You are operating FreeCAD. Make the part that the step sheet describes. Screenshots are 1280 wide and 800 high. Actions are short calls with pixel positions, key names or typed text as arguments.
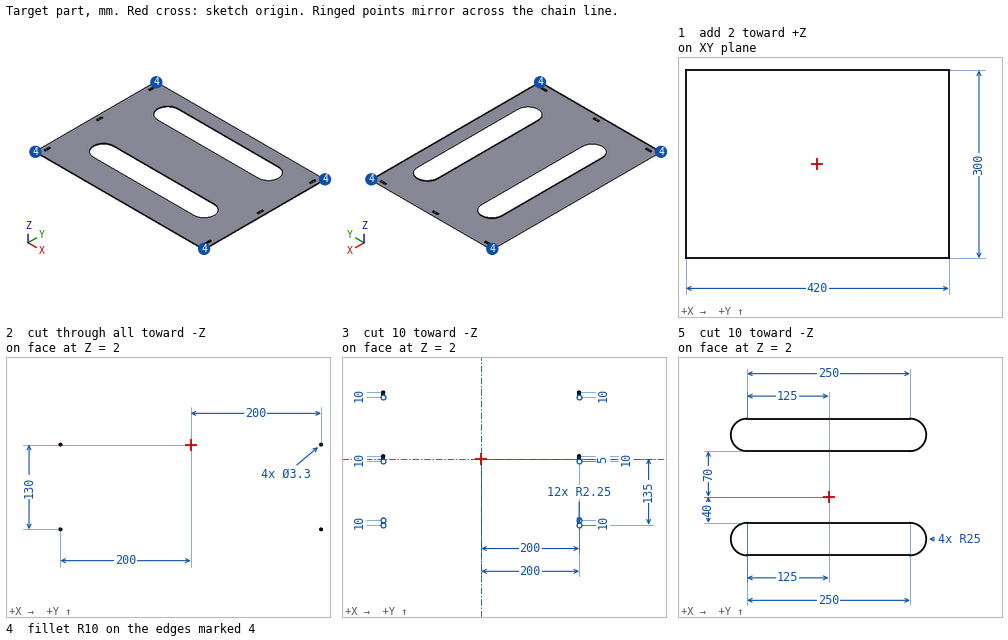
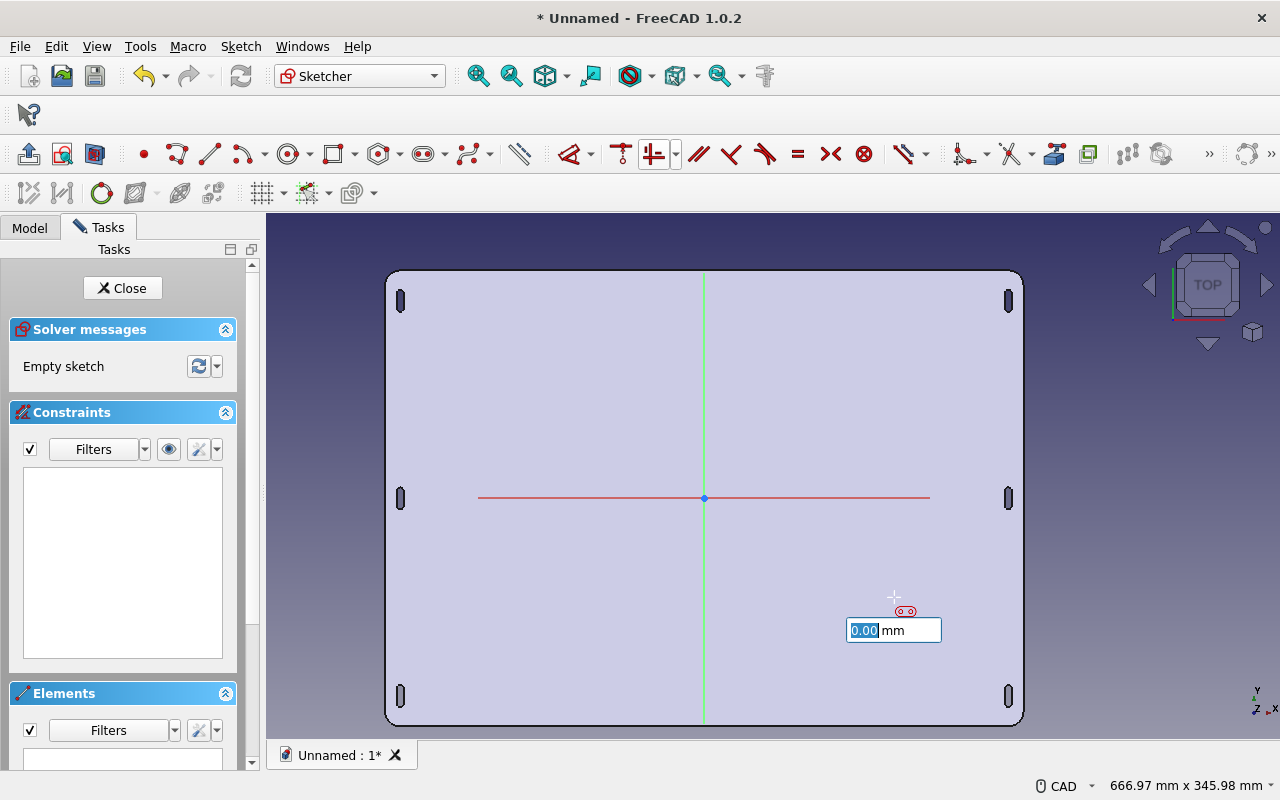
click(761, 559)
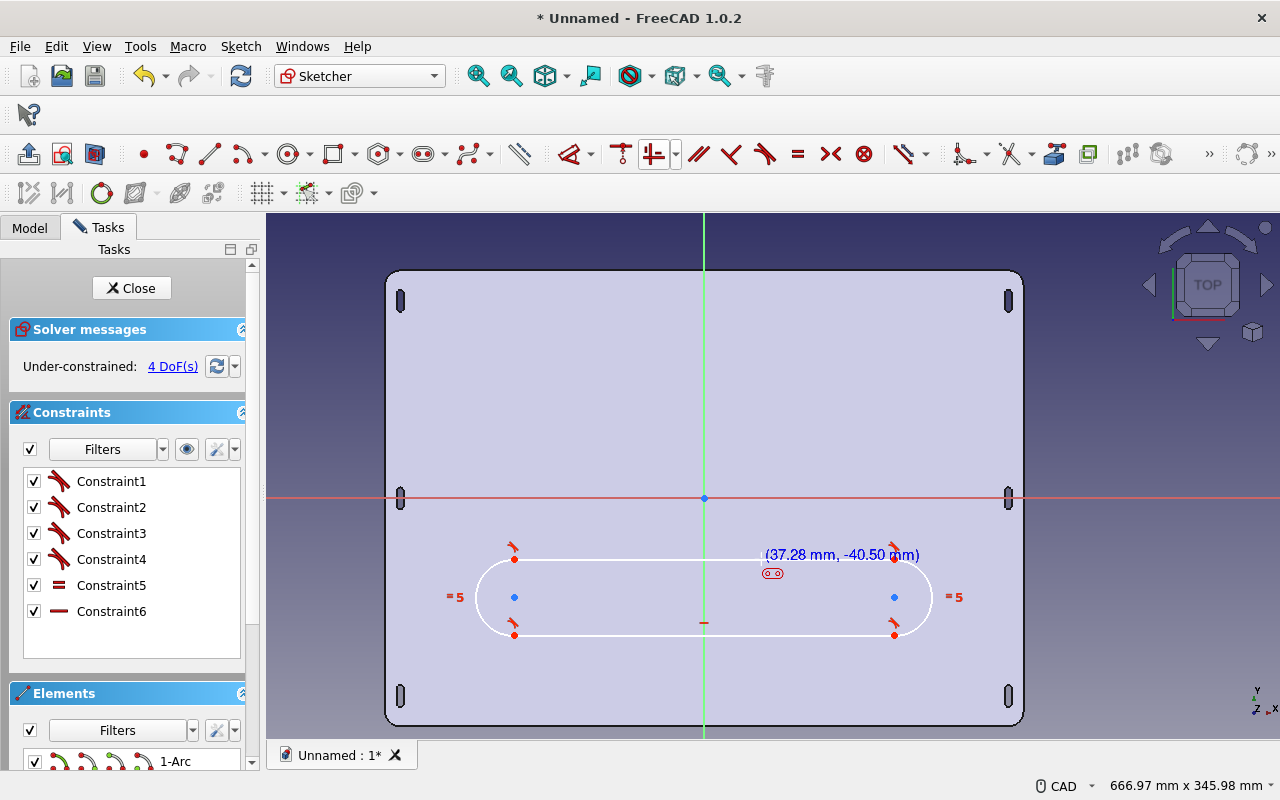
click(514, 354)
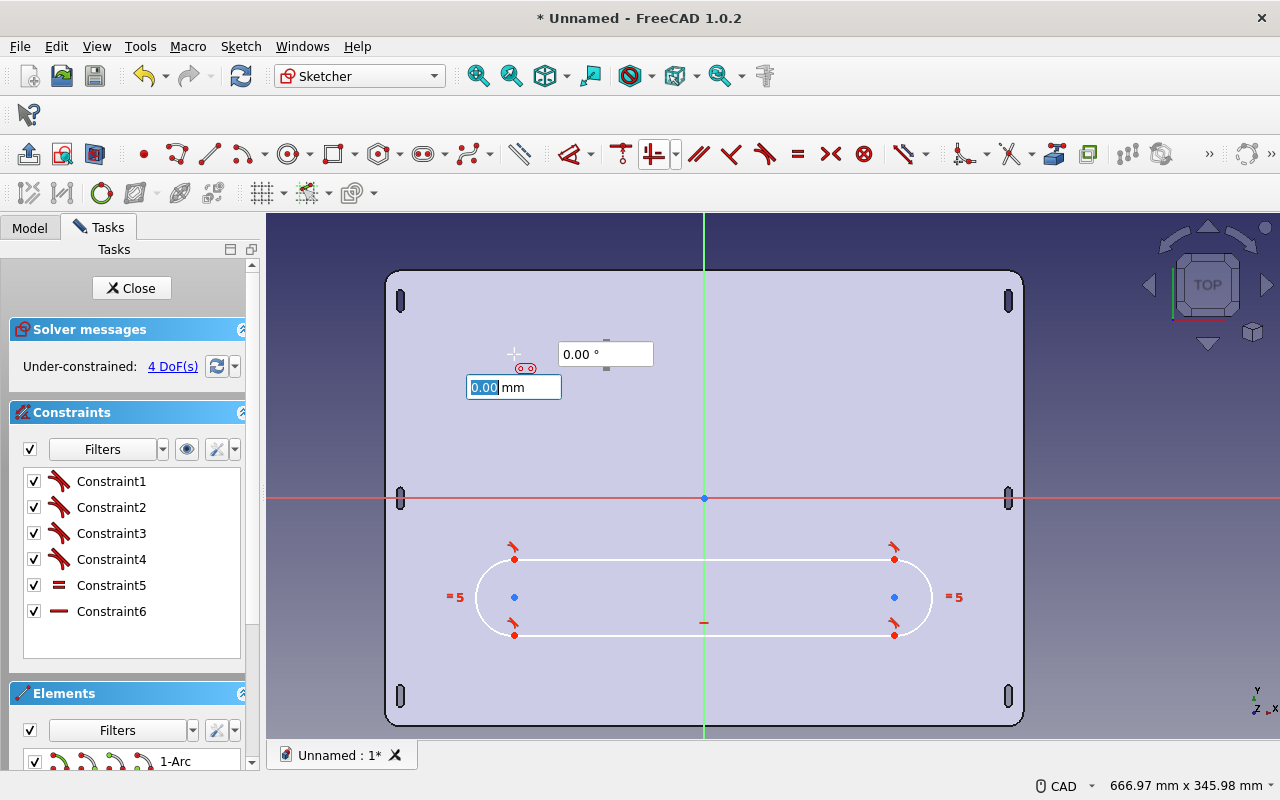
click(894, 354)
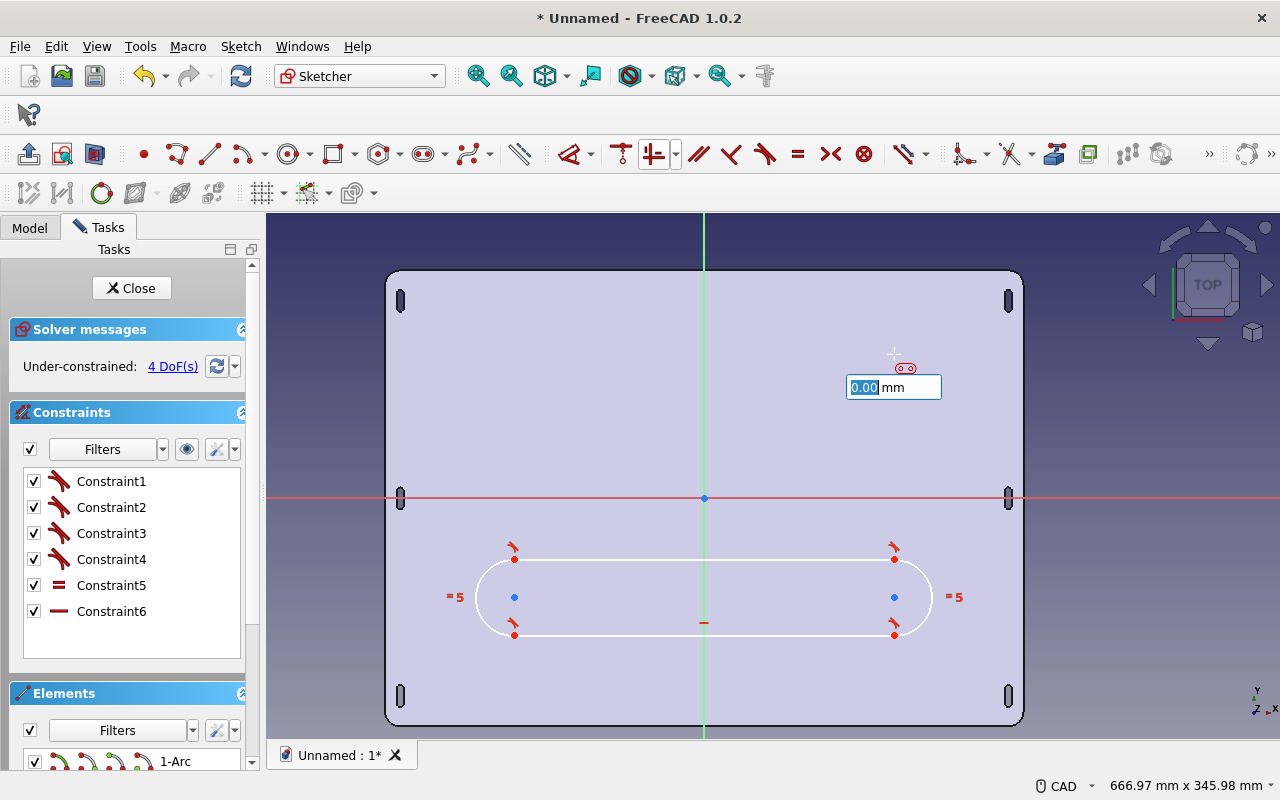
click(647, 392)
key(Escape)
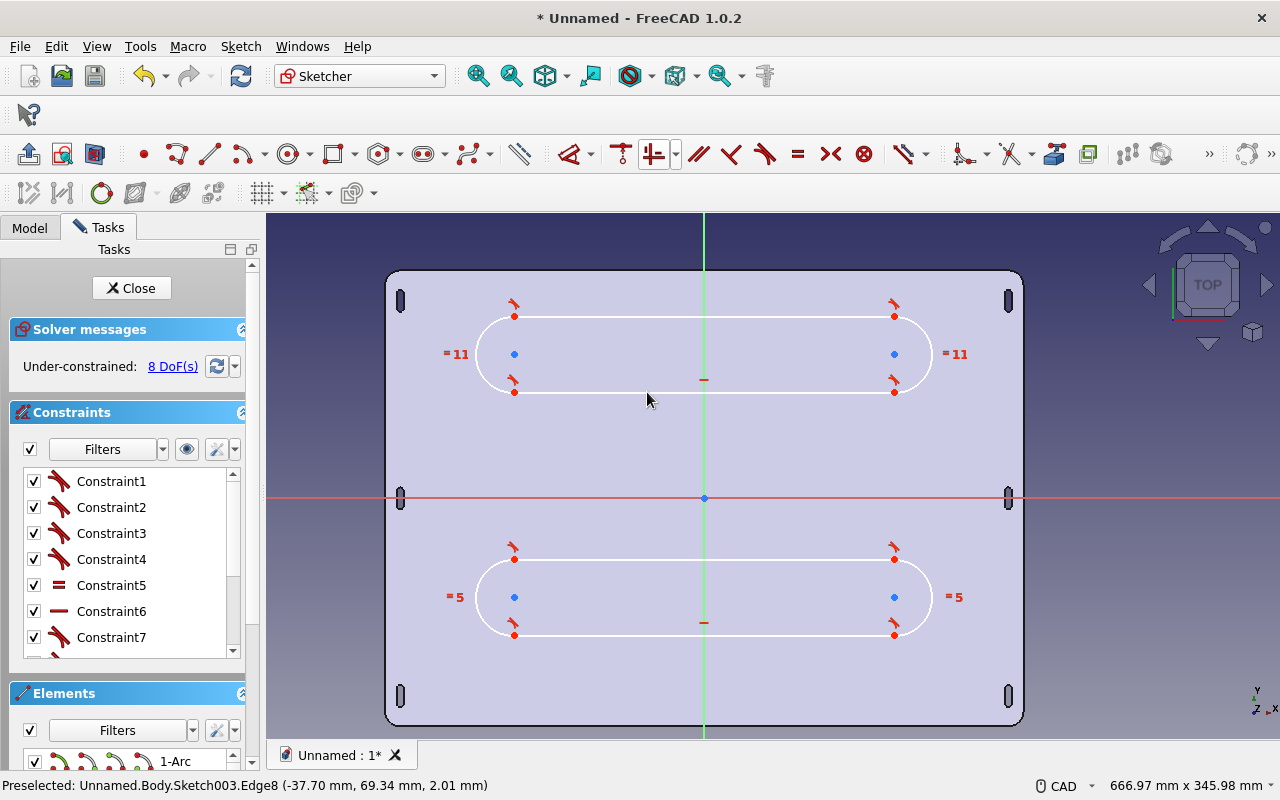
click(483, 576)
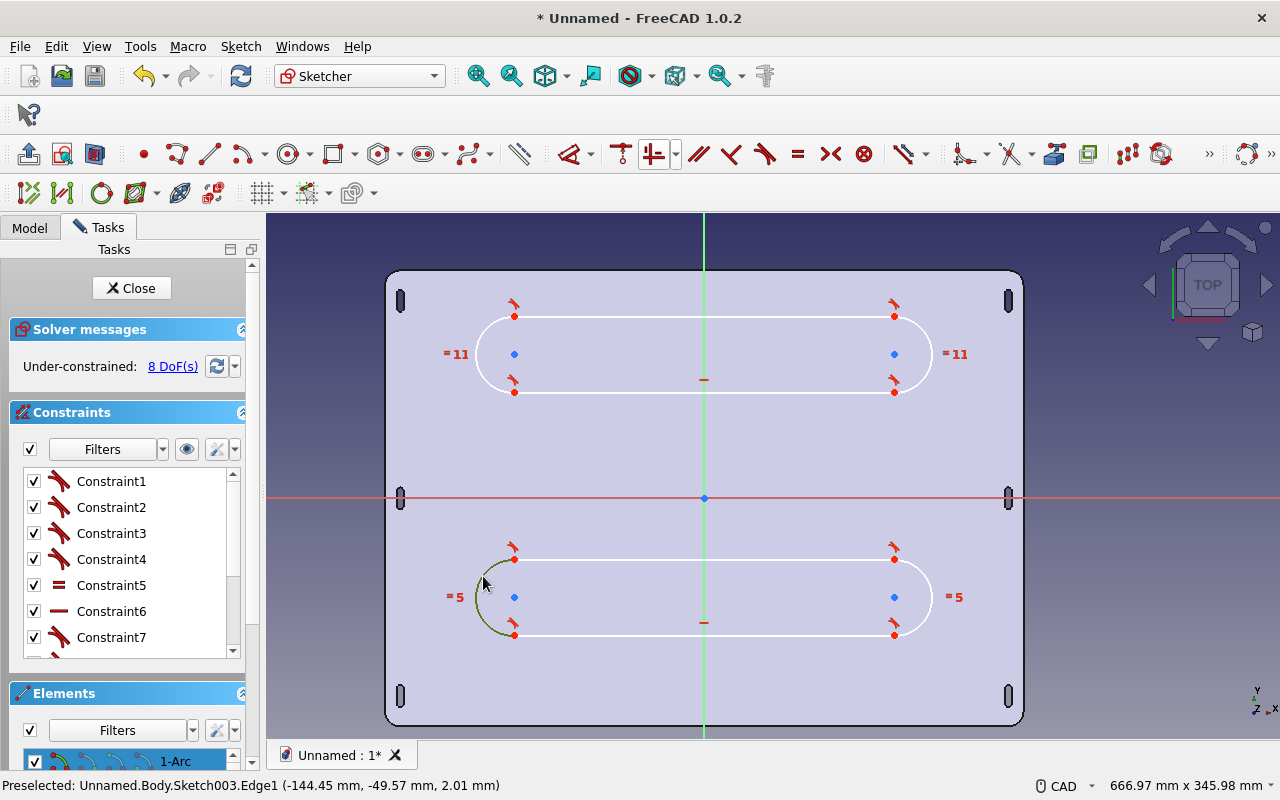
click(483, 333)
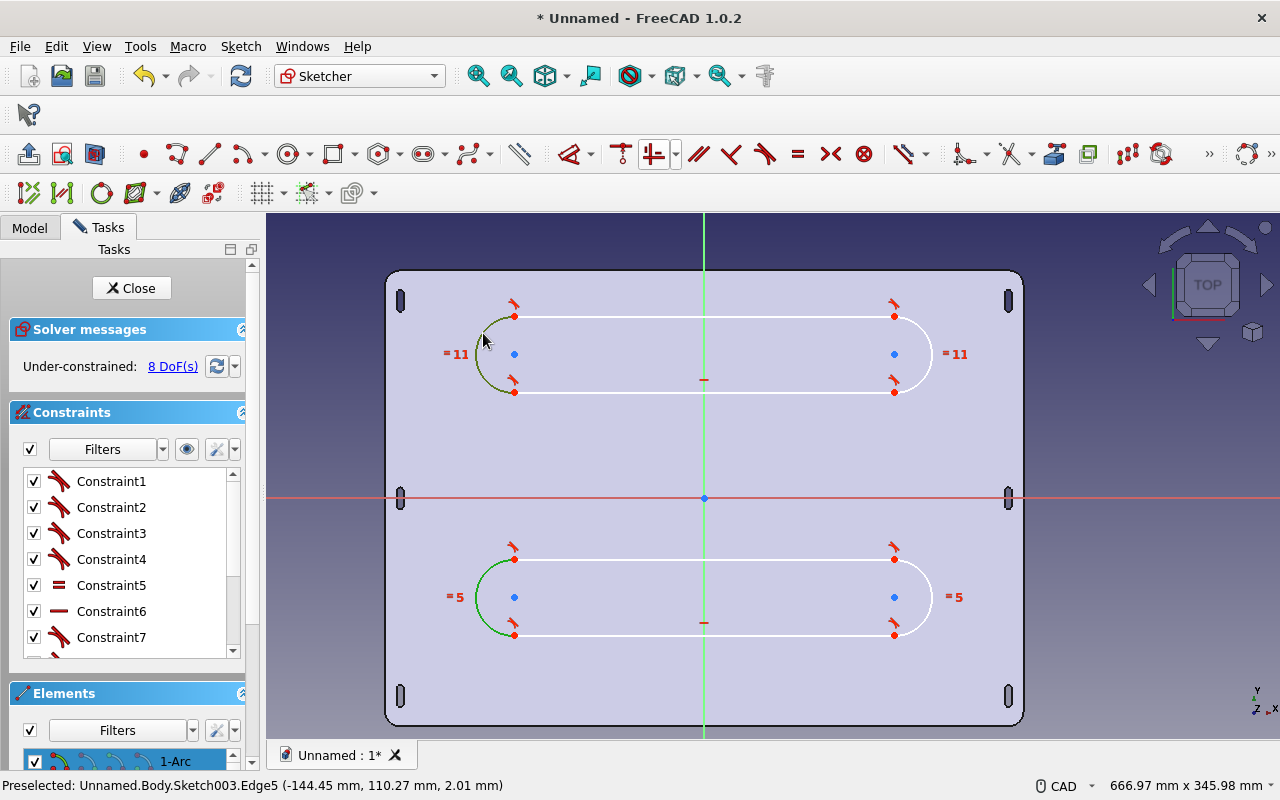
click(798, 154)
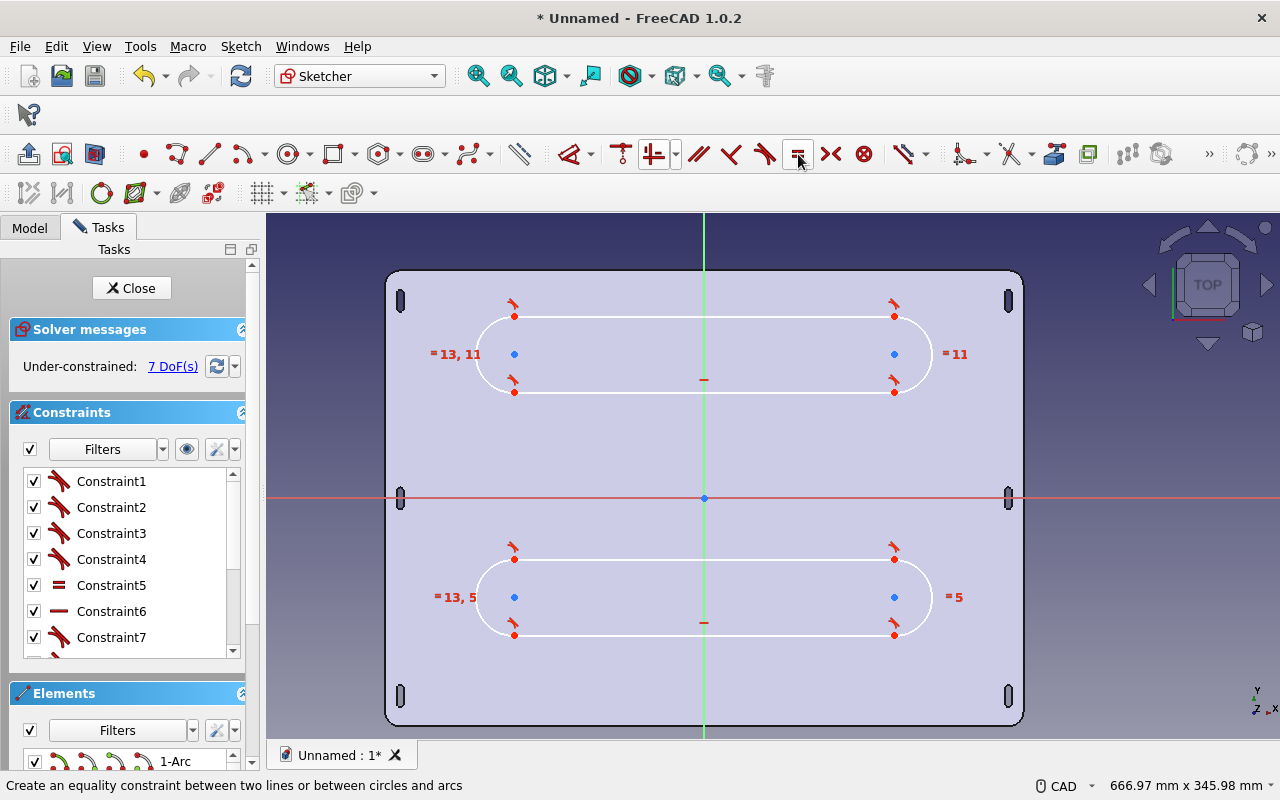
key(d)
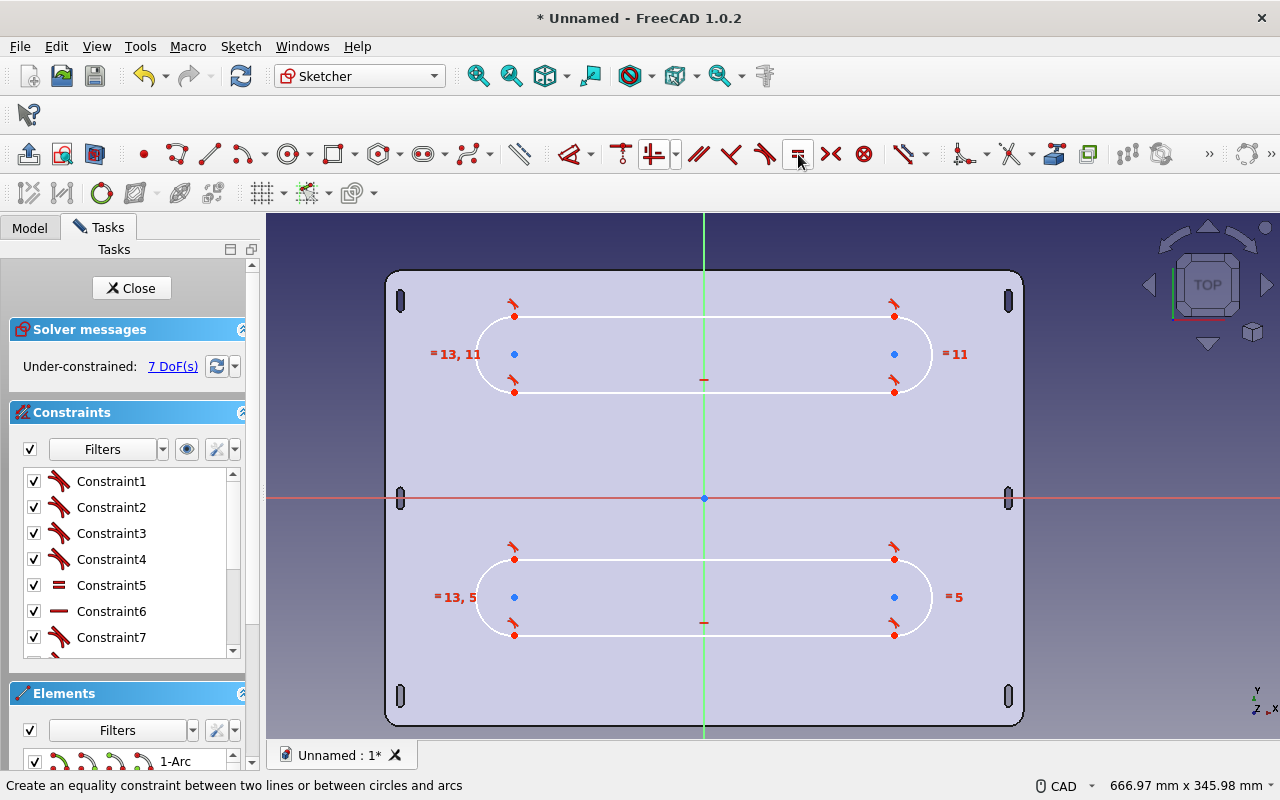
click(483, 576)
click(457, 557)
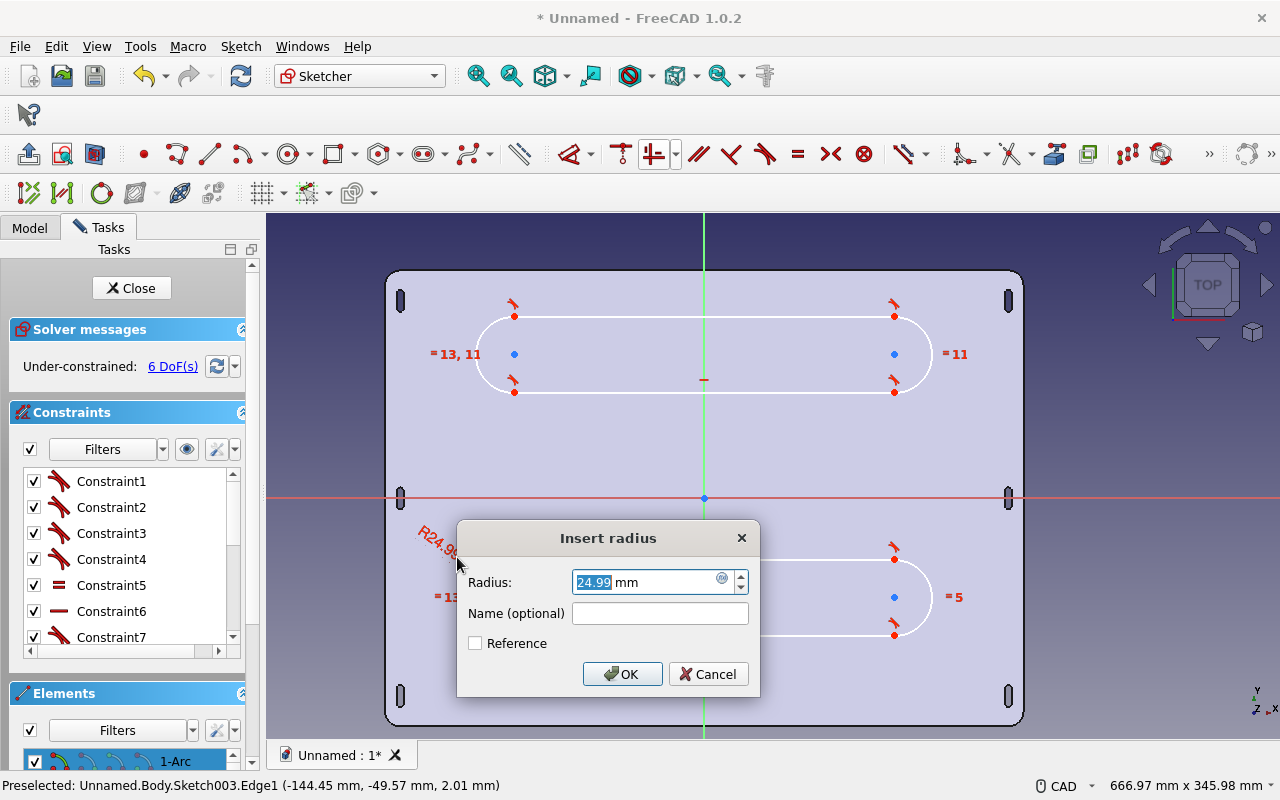
text(25)
key(Return)